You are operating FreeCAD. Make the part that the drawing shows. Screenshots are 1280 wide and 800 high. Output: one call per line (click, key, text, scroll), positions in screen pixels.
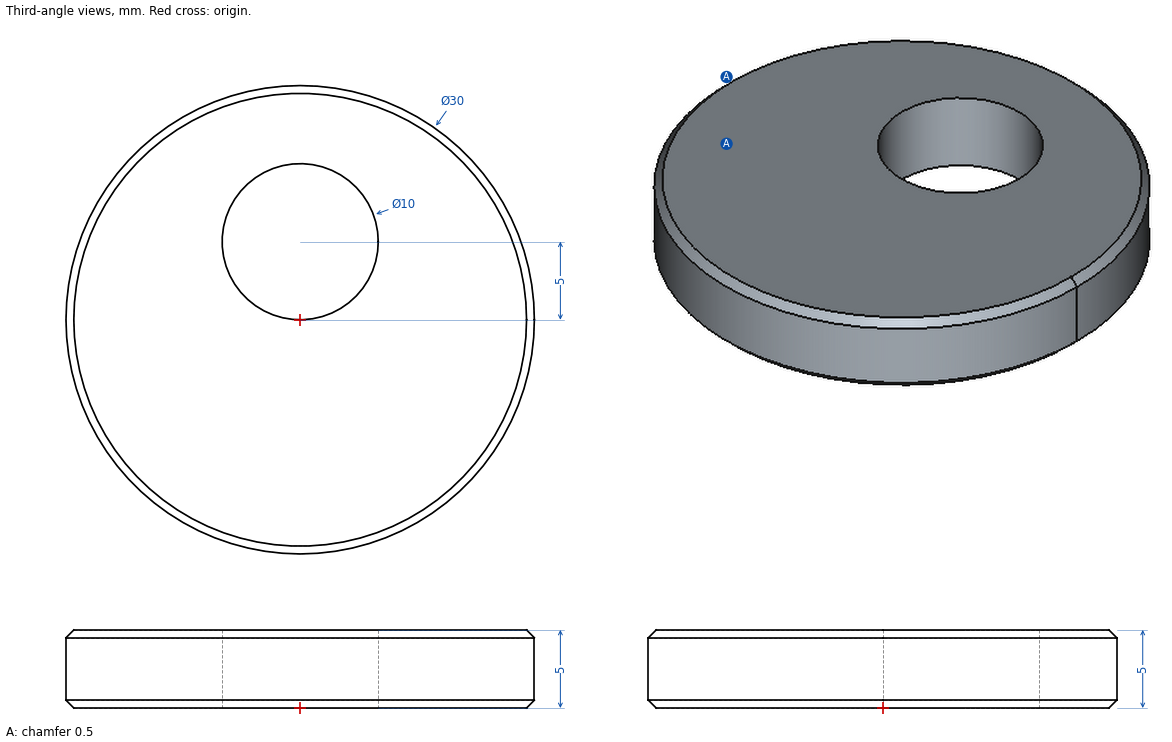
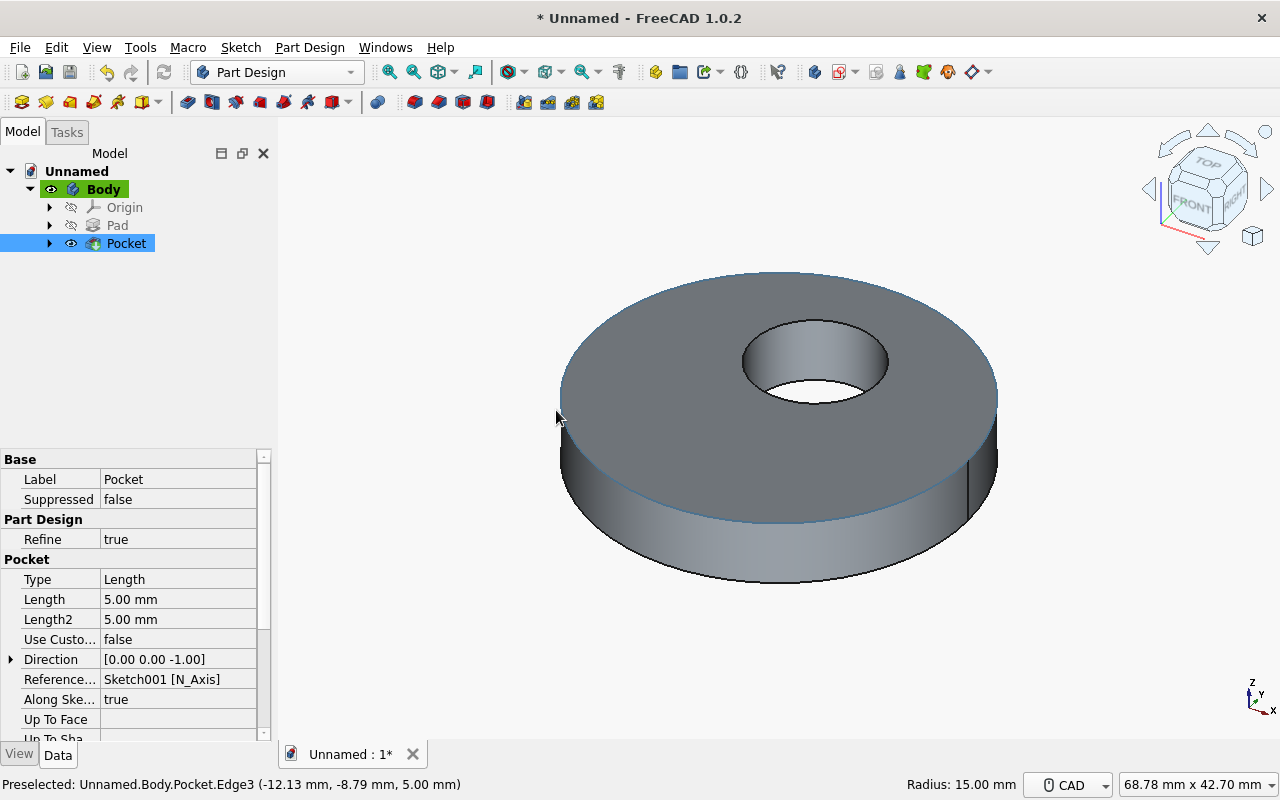
key(0)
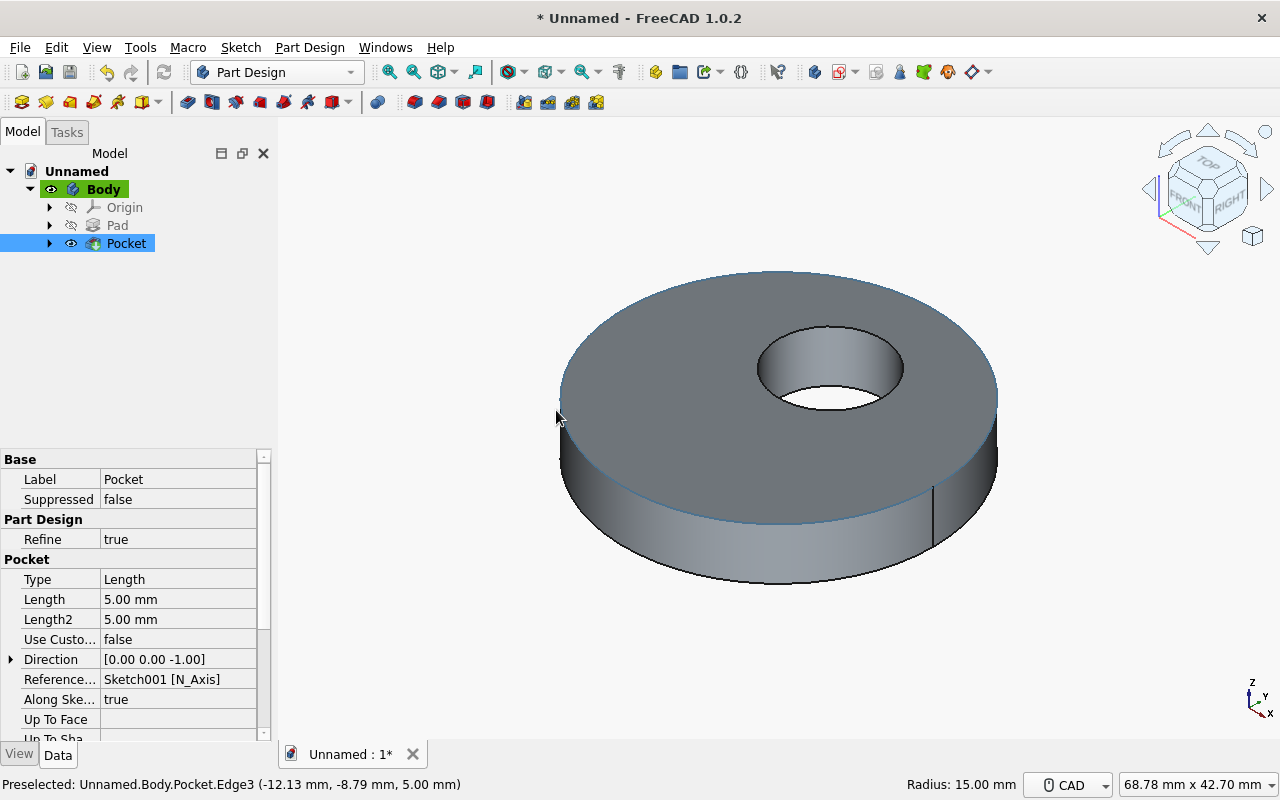
key(2)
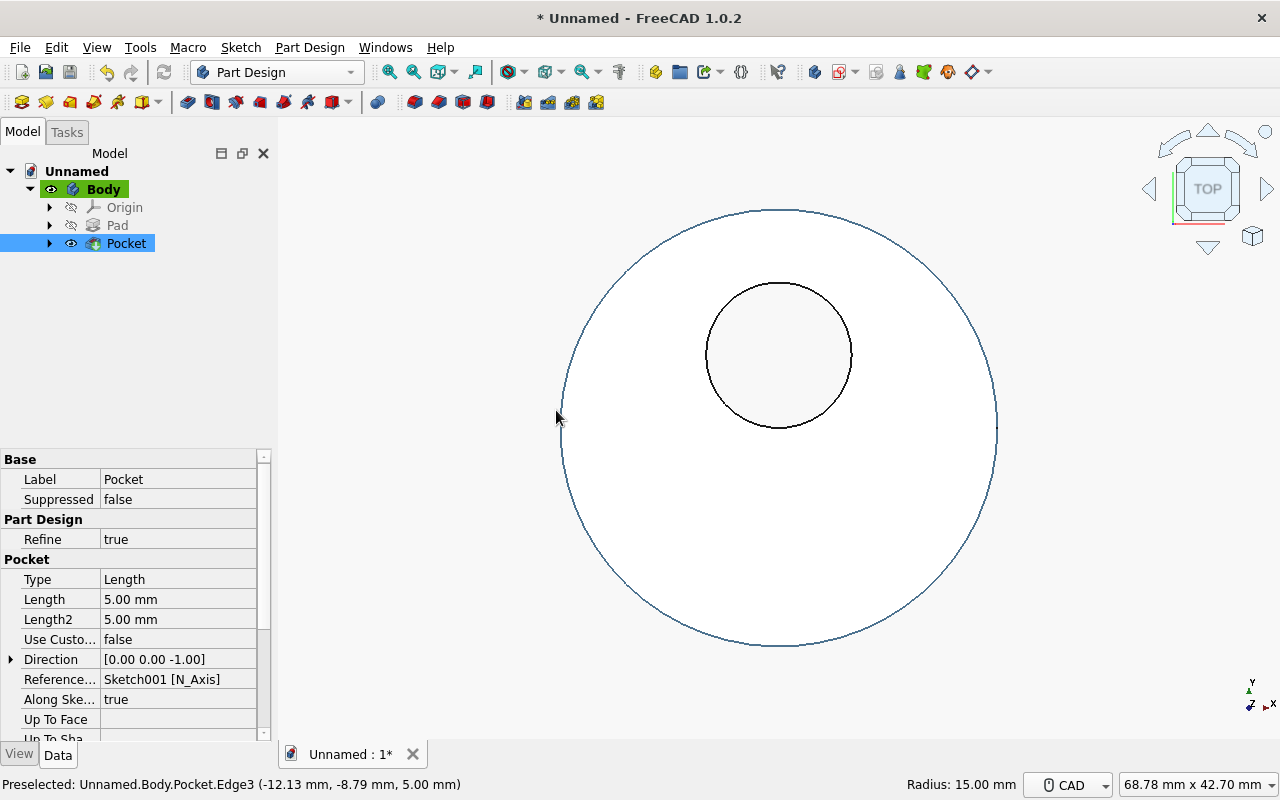
key(1)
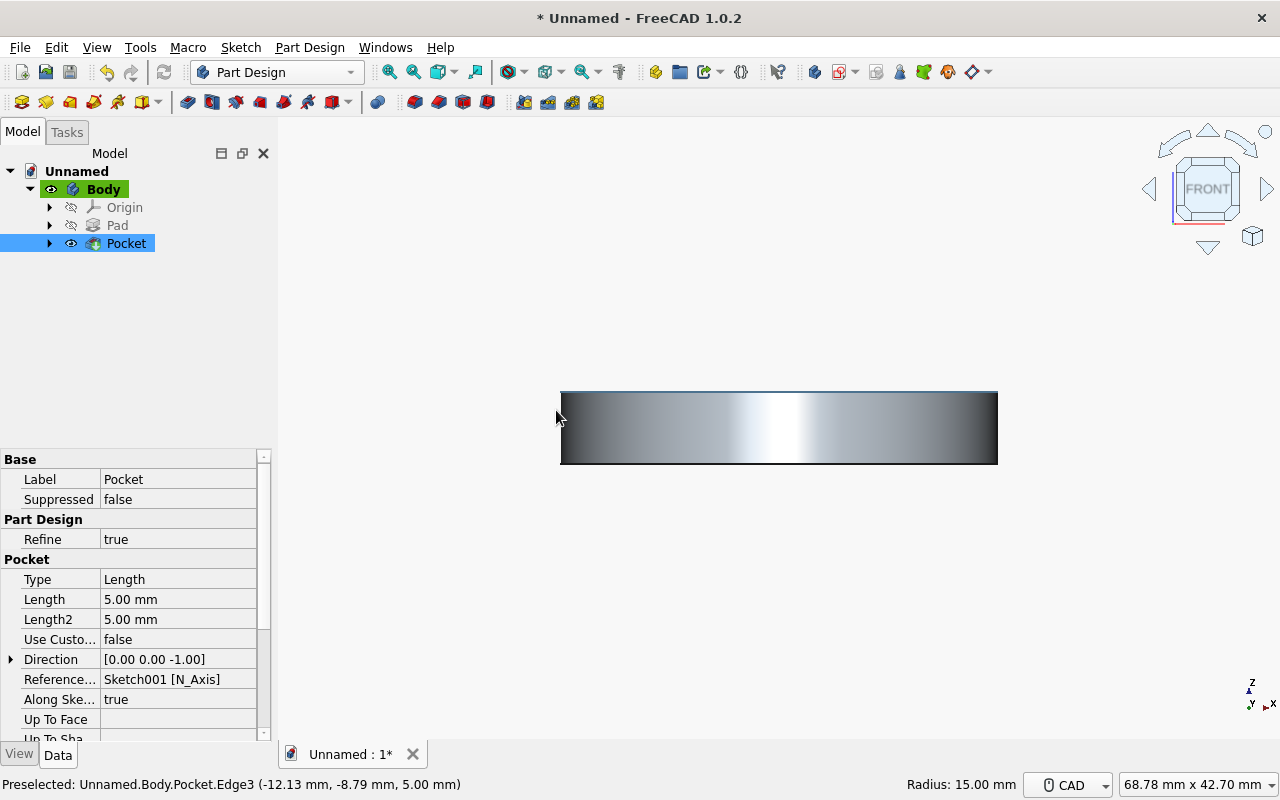
key(v)
key(f)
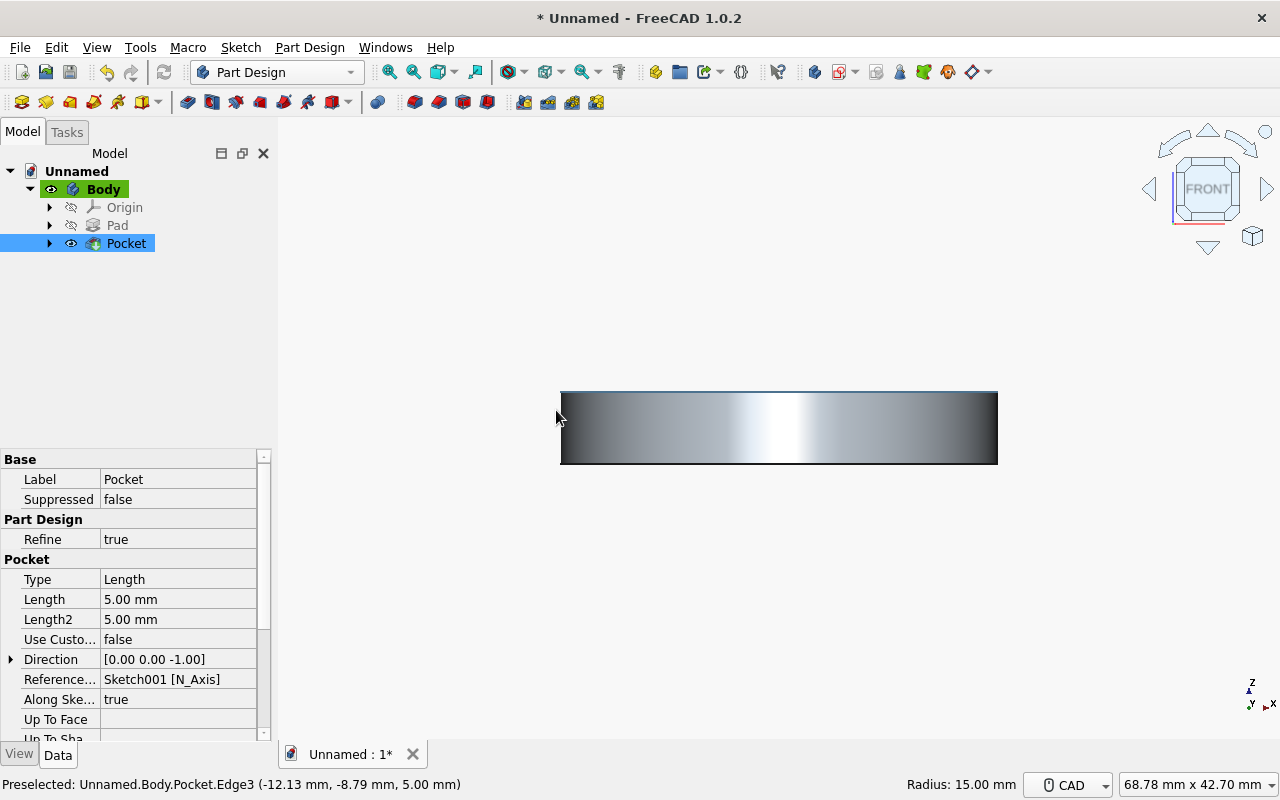
click(602, 463, ctrl)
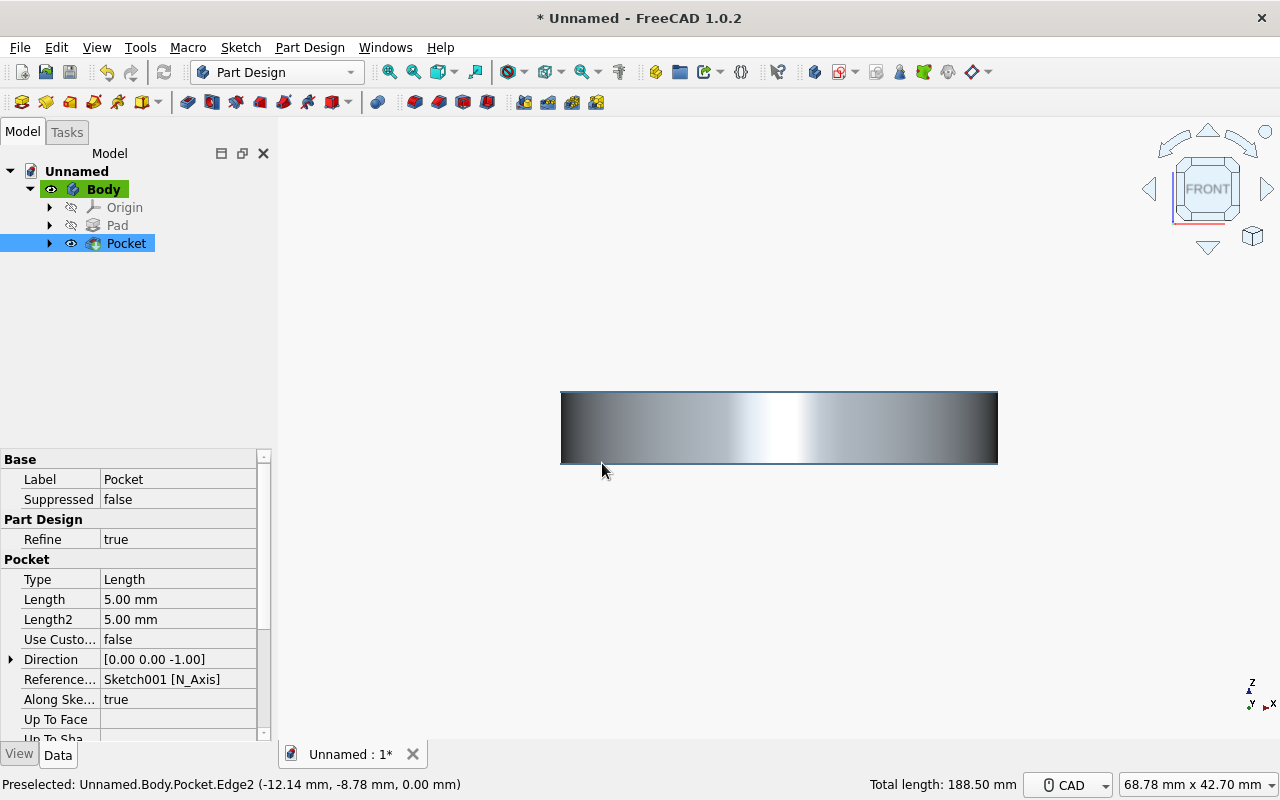
click(440, 102)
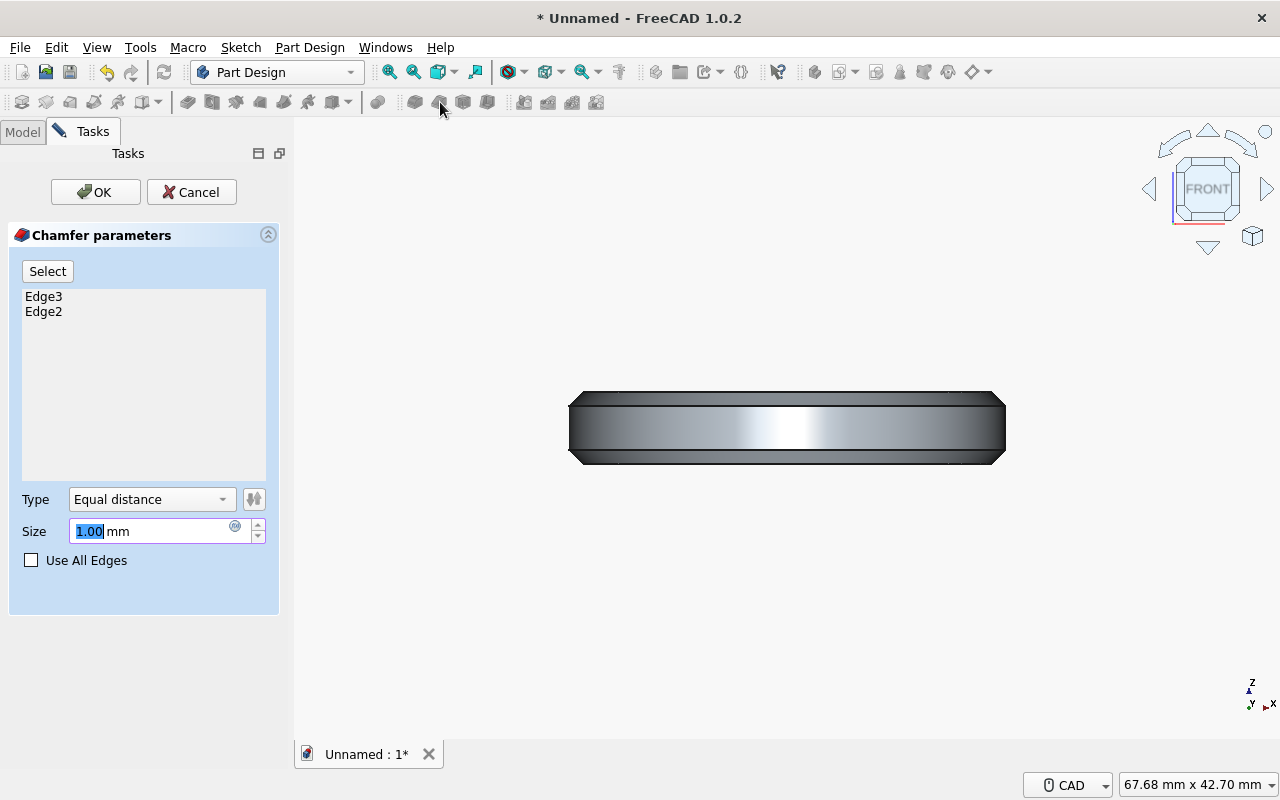
text(0.5)
key(Tab)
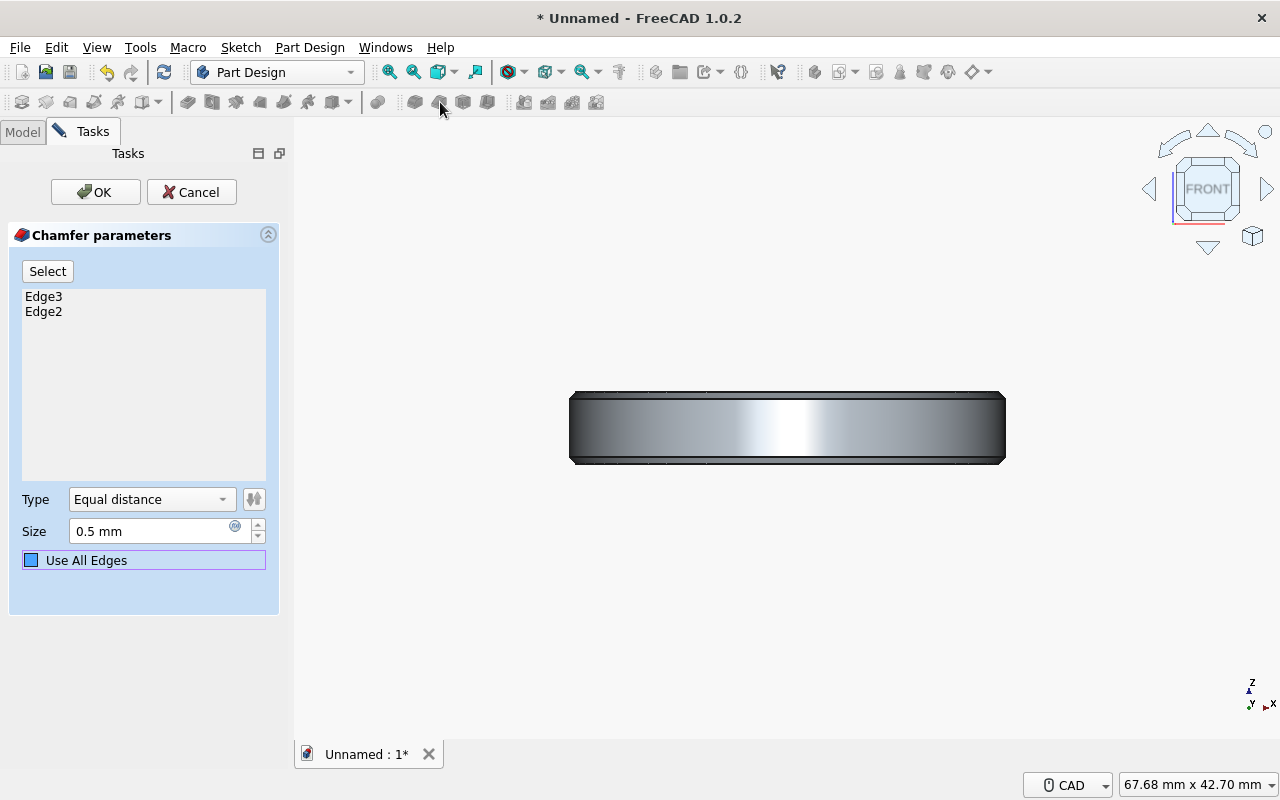
click(96, 192)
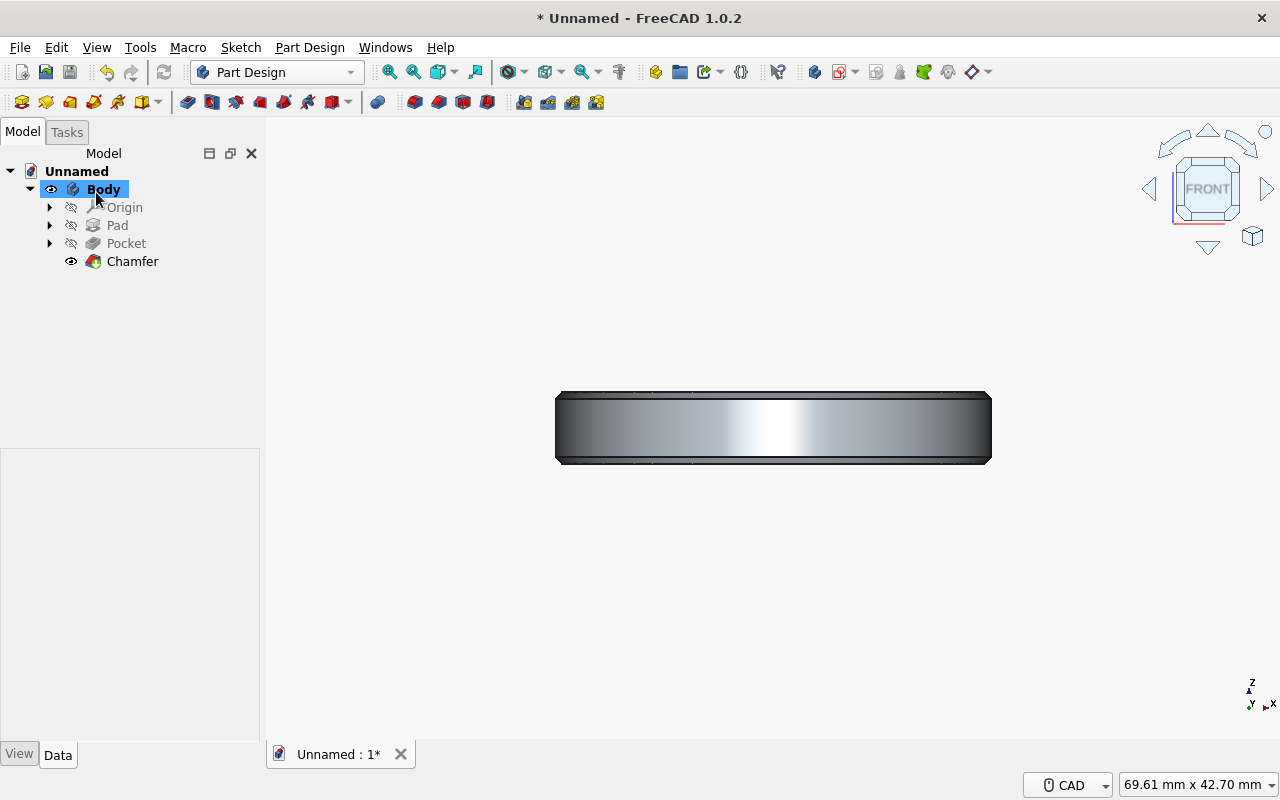
key(0)